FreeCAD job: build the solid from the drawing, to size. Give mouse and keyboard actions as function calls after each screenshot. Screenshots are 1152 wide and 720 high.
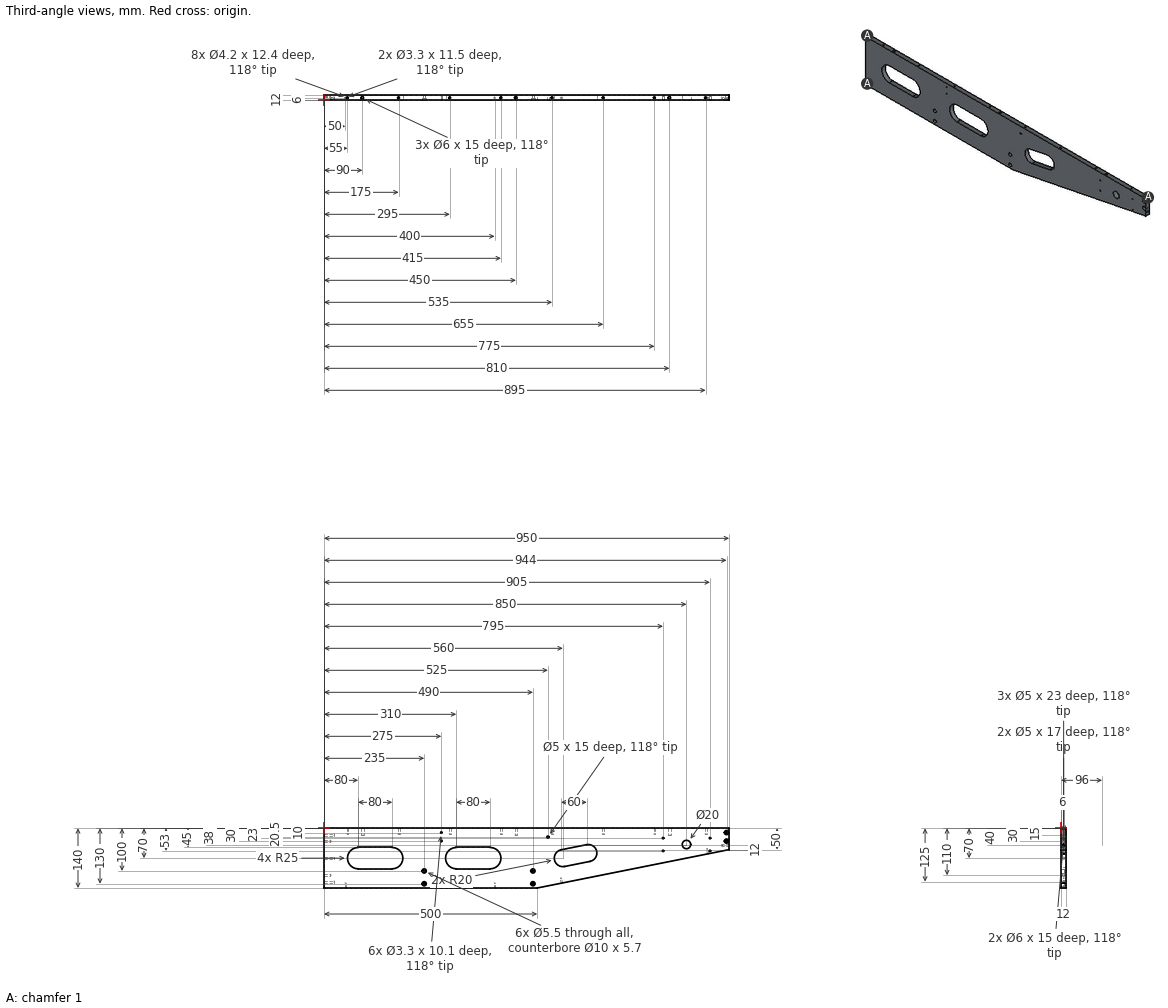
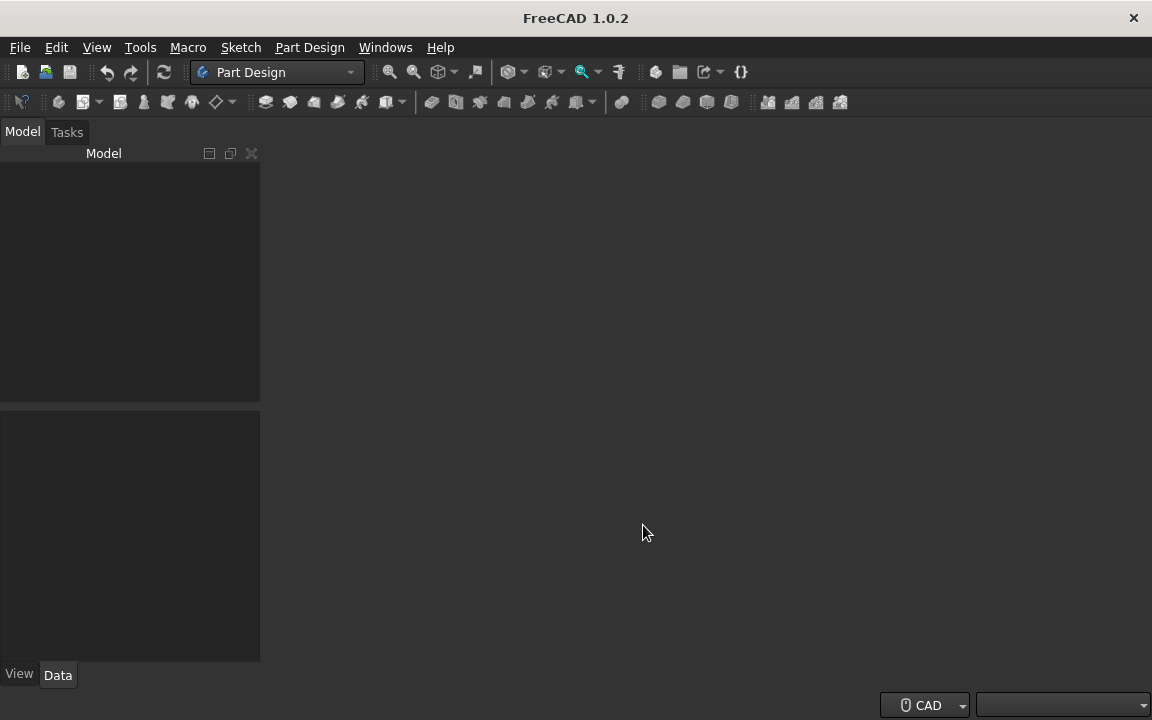
key(ctrl+n)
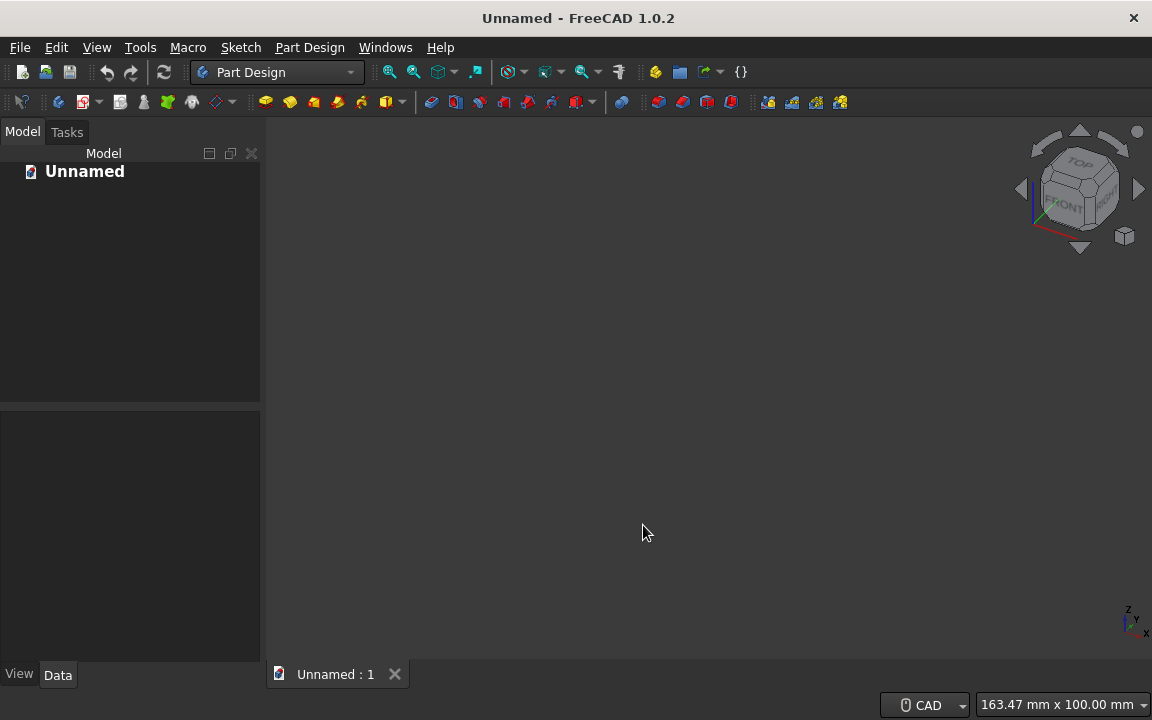
click(84, 102)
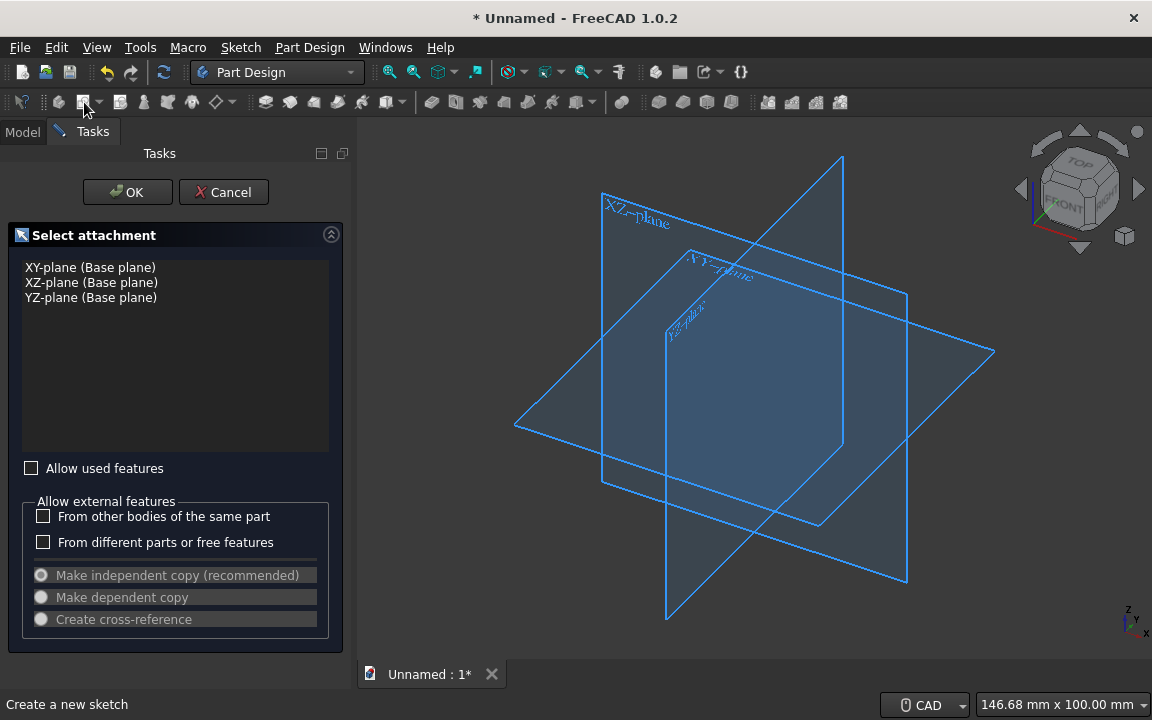
click(82, 282)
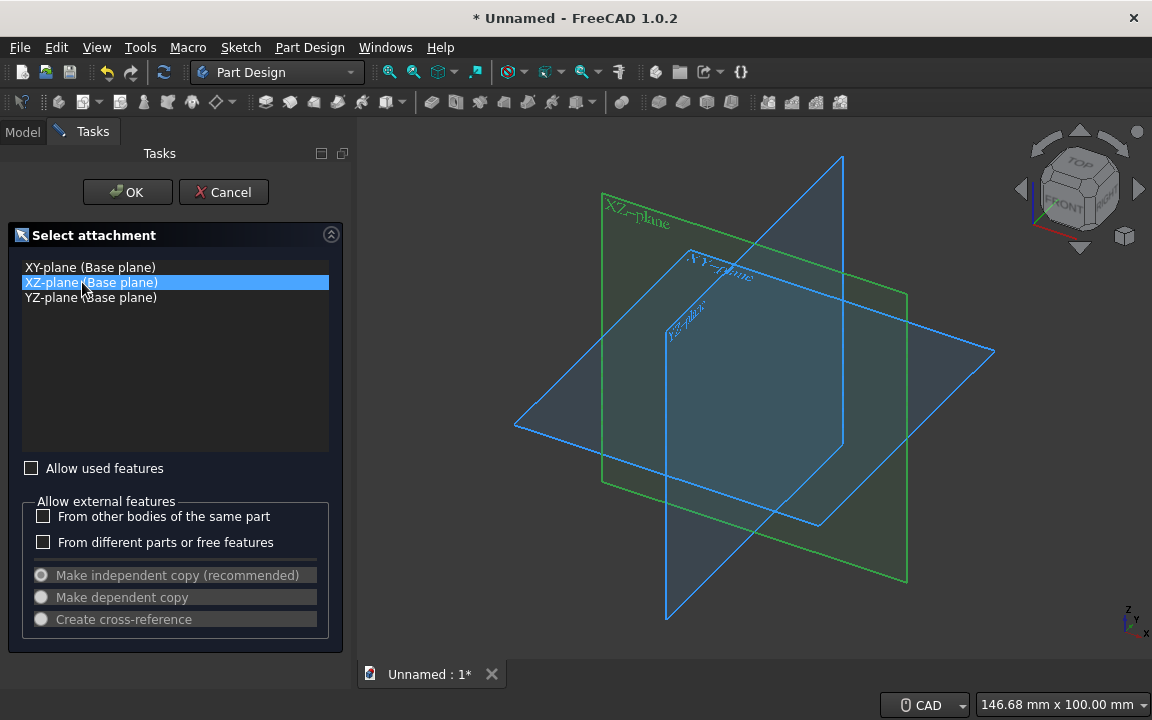
click(128, 192)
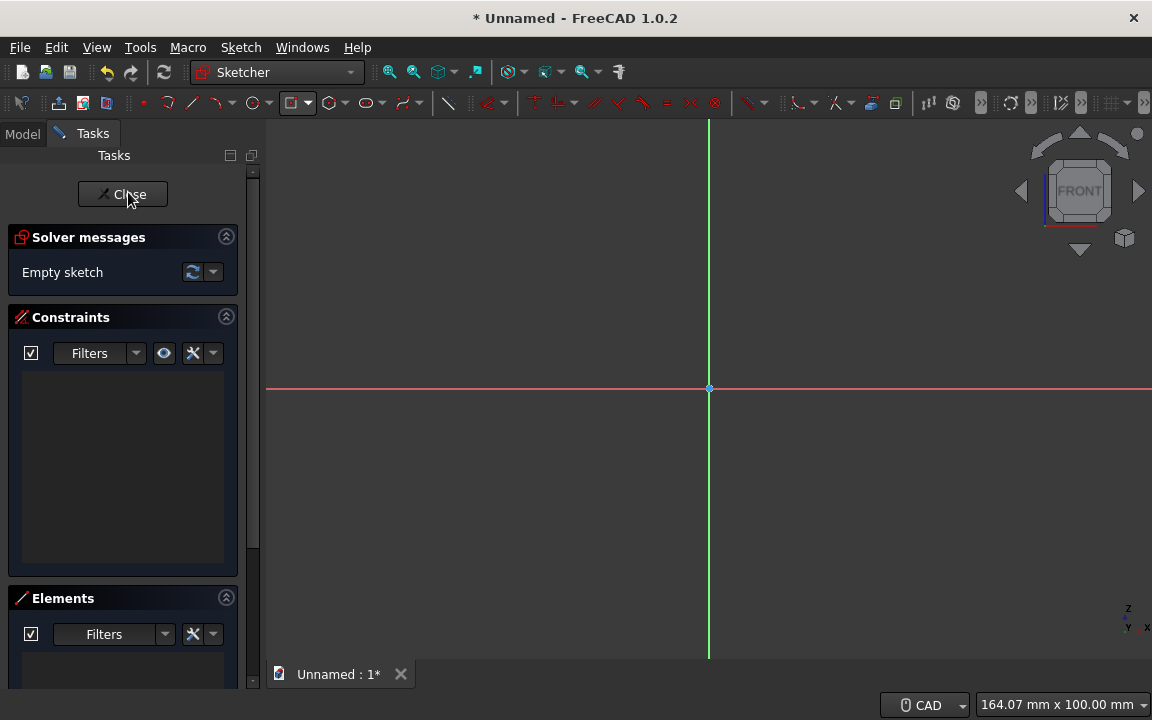
scroll(378, 351, down, 12)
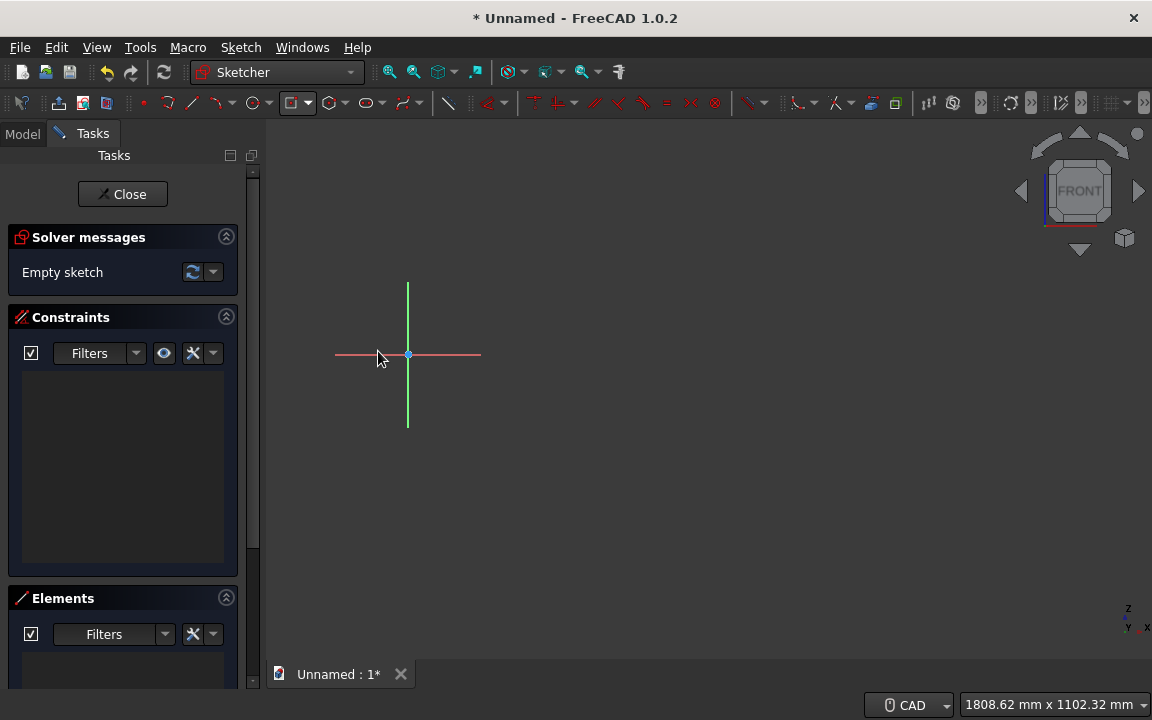
key(g)
key(m)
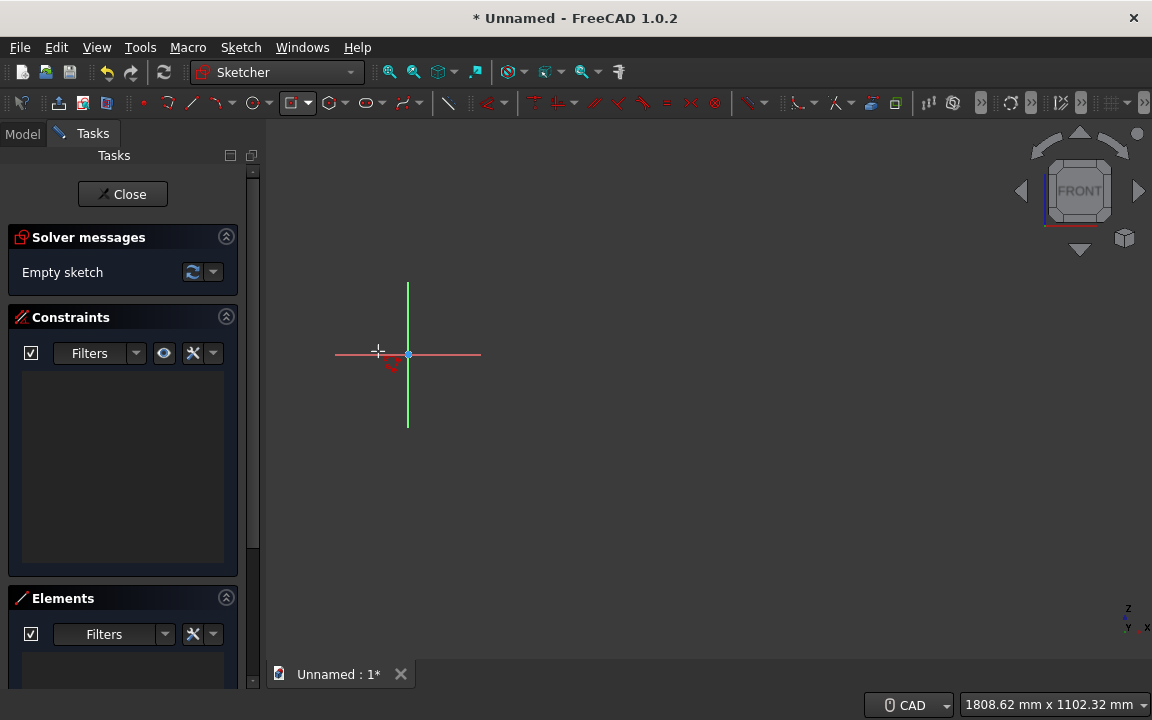
click(408, 355)
click(417, 423)
click(653, 423)
click(874, 379)
click(874, 364)
click(408, 355)
key(Escape)
key(Escape)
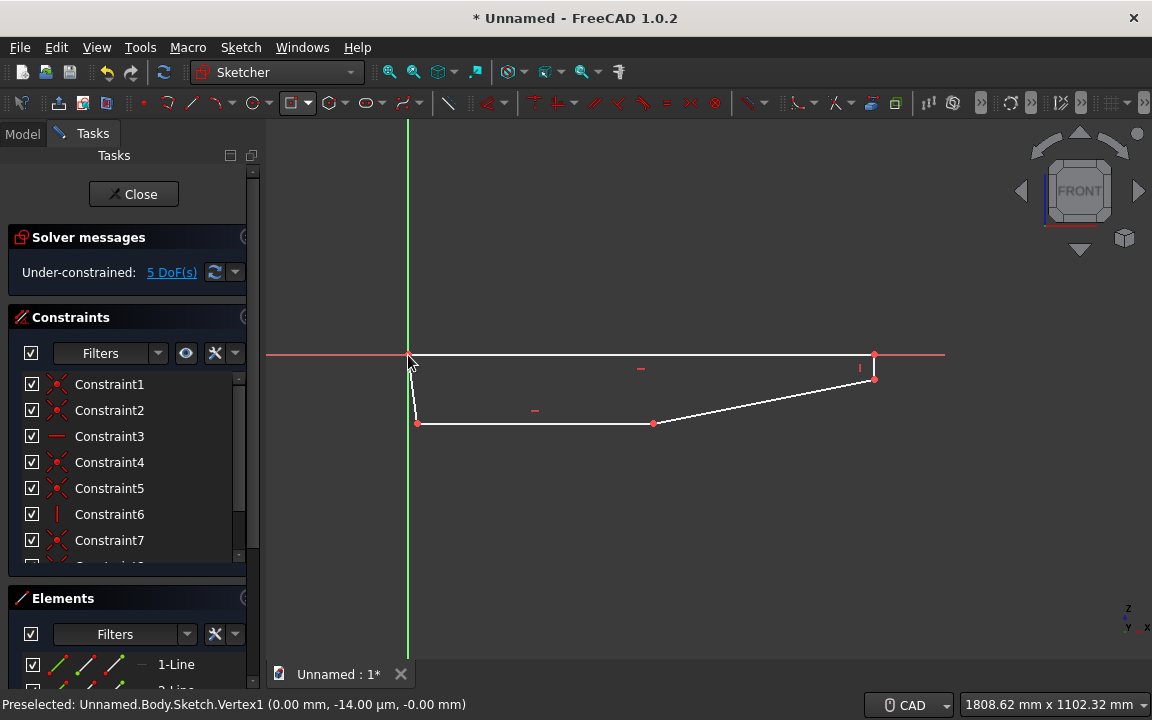
click(411, 376)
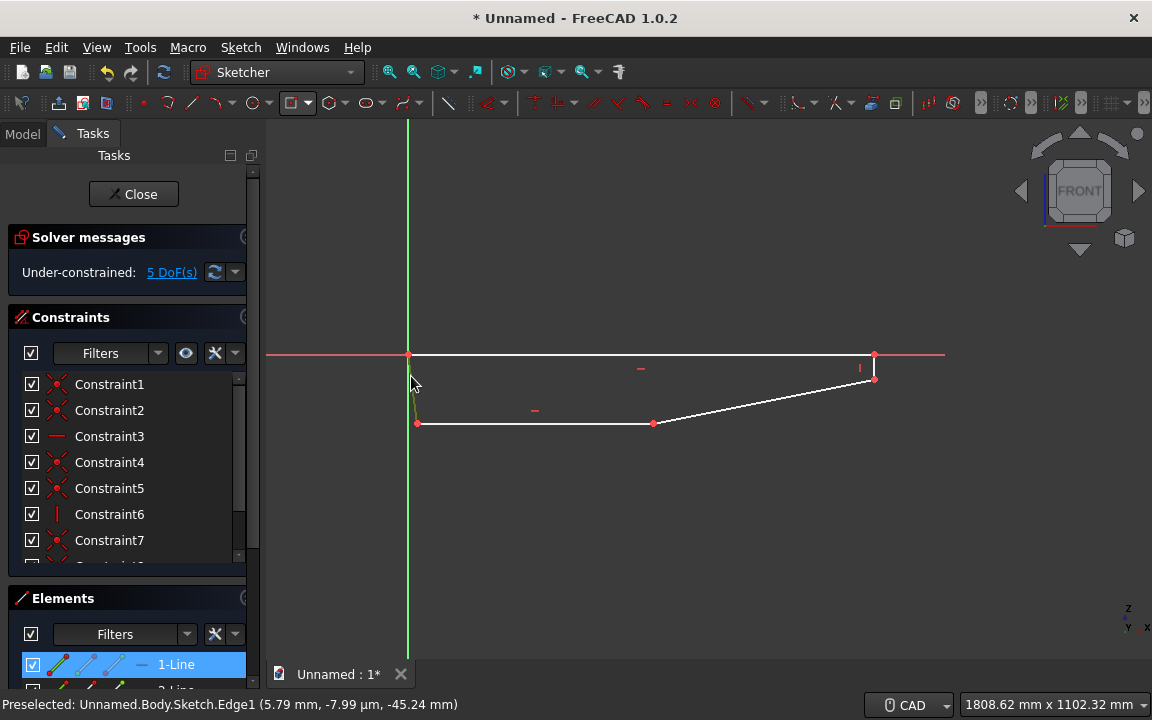
key(v)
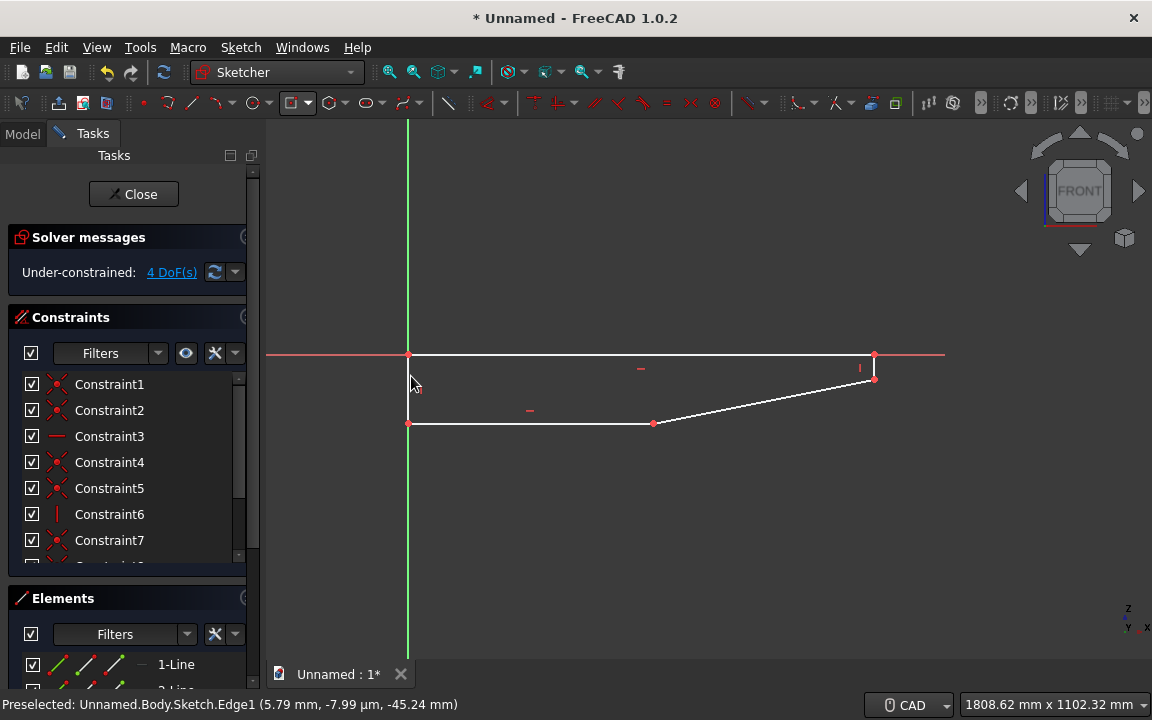
scroll(874, 370, up, 3)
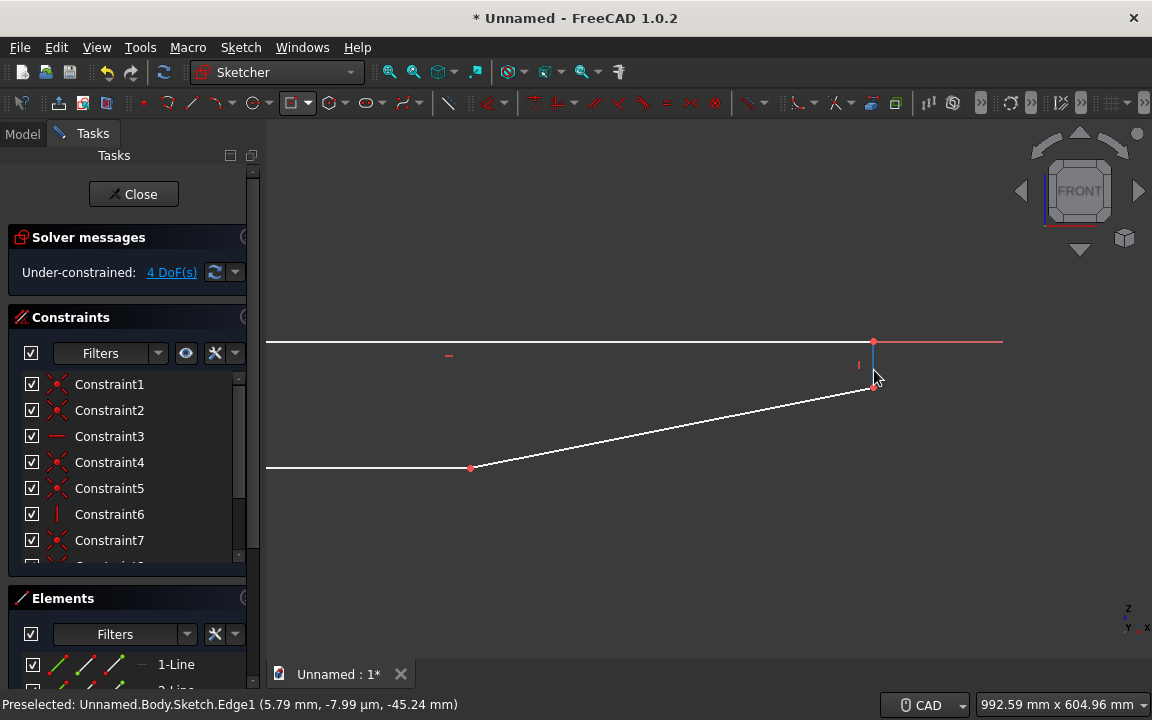
click(873, 369)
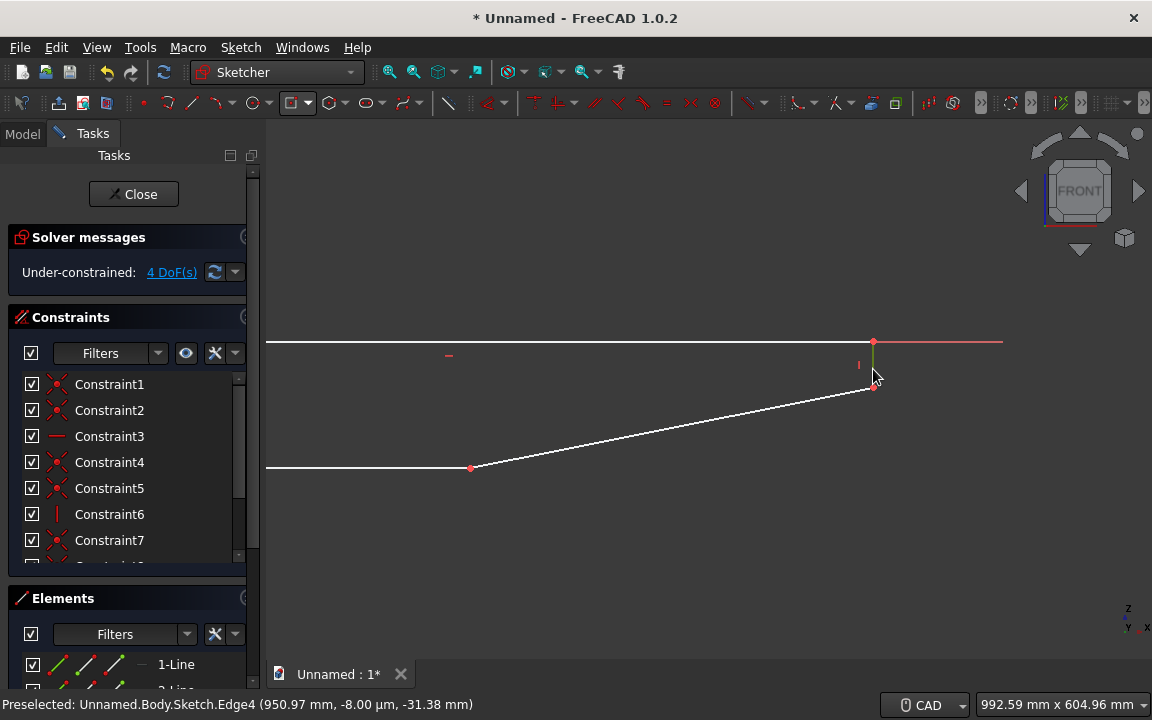
key(i)